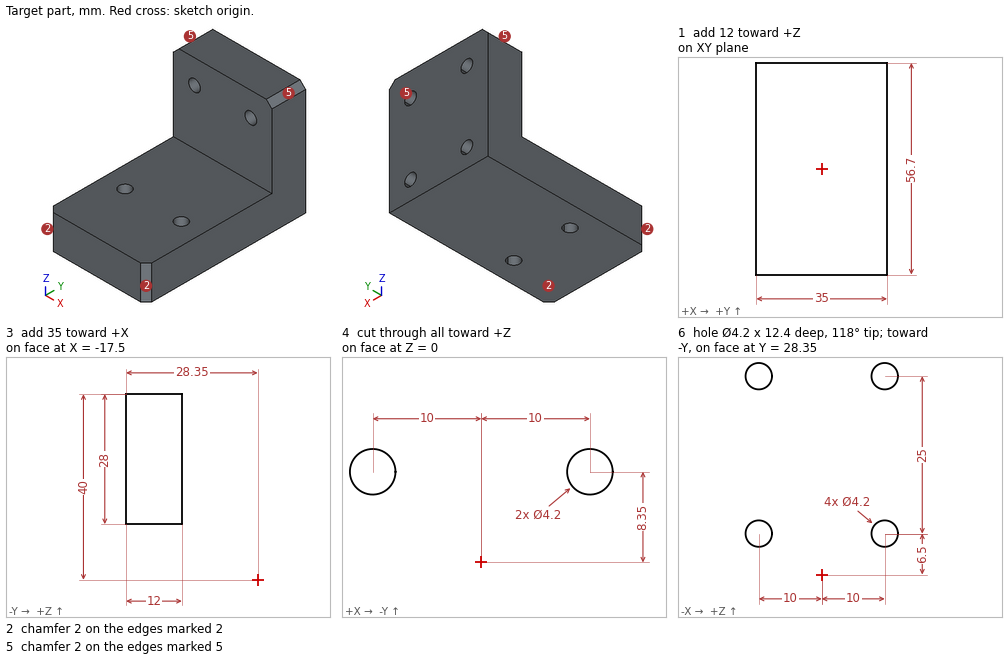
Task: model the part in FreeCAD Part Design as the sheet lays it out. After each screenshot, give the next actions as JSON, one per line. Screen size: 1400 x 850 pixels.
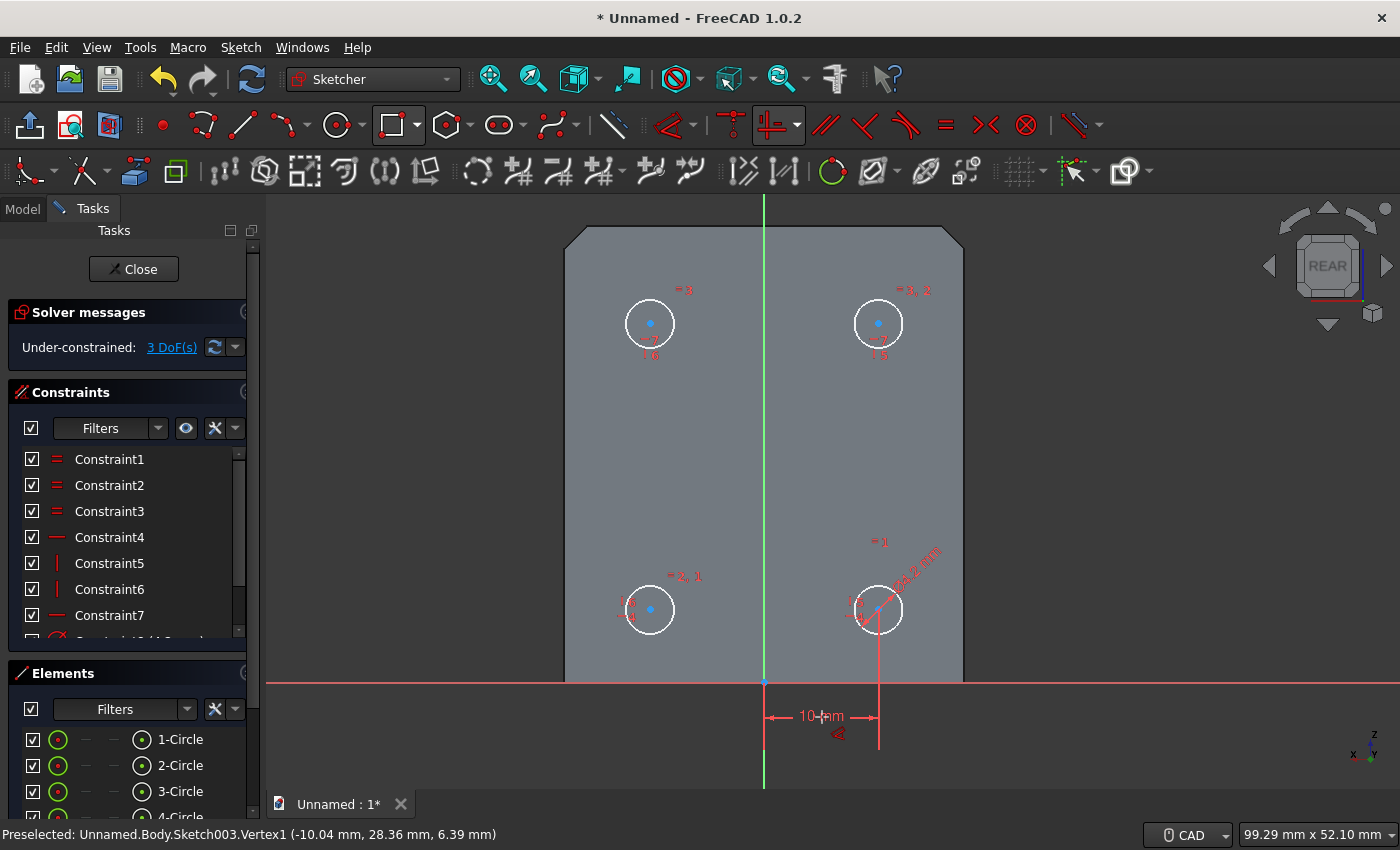
{"action": "left_click", "coordinate": [650, 610]}
{"action": "left_click", "coordinate": [707, 717]}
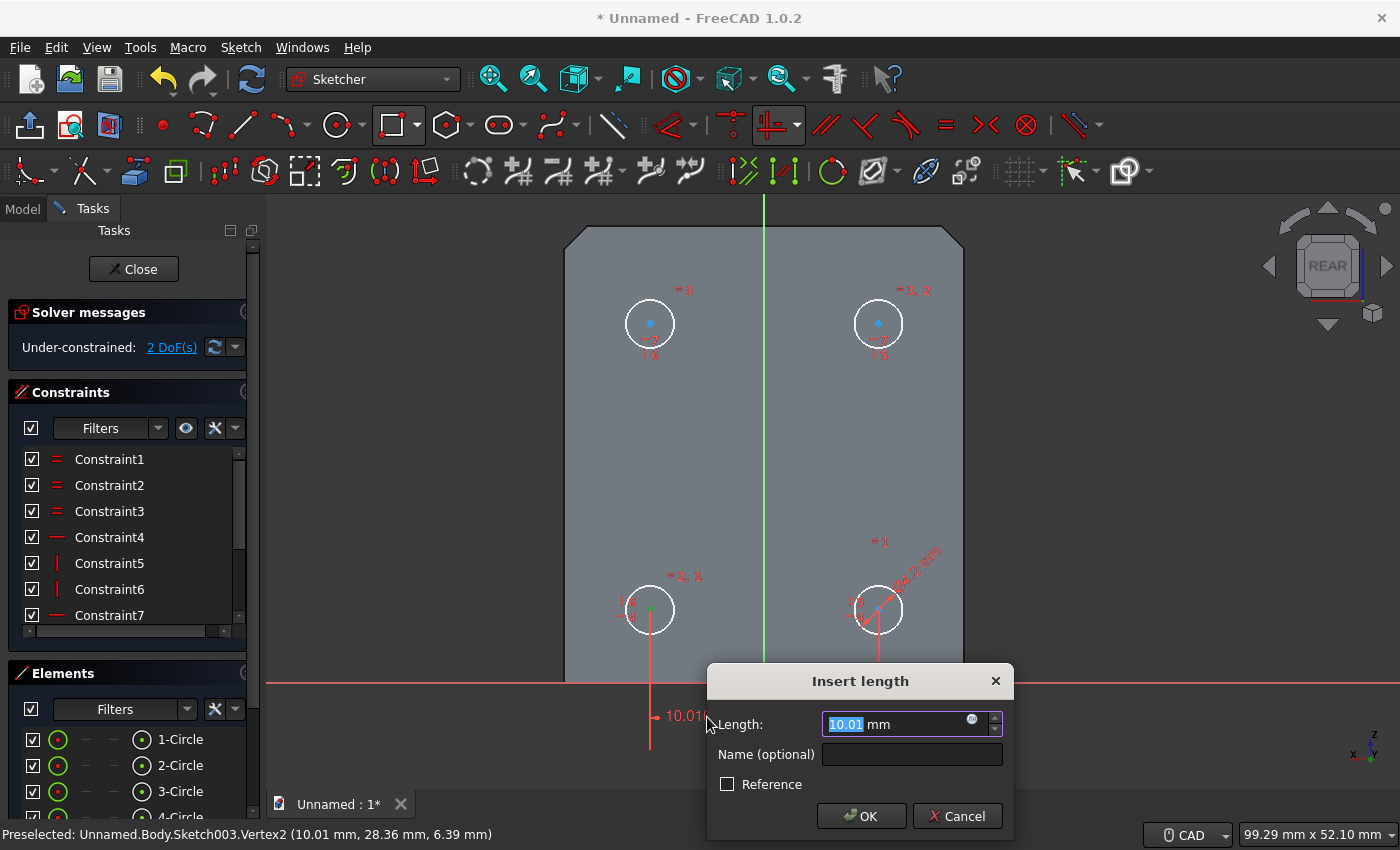
{"action": "type", "text": "10"}
{"action": "key", "text": "Return"}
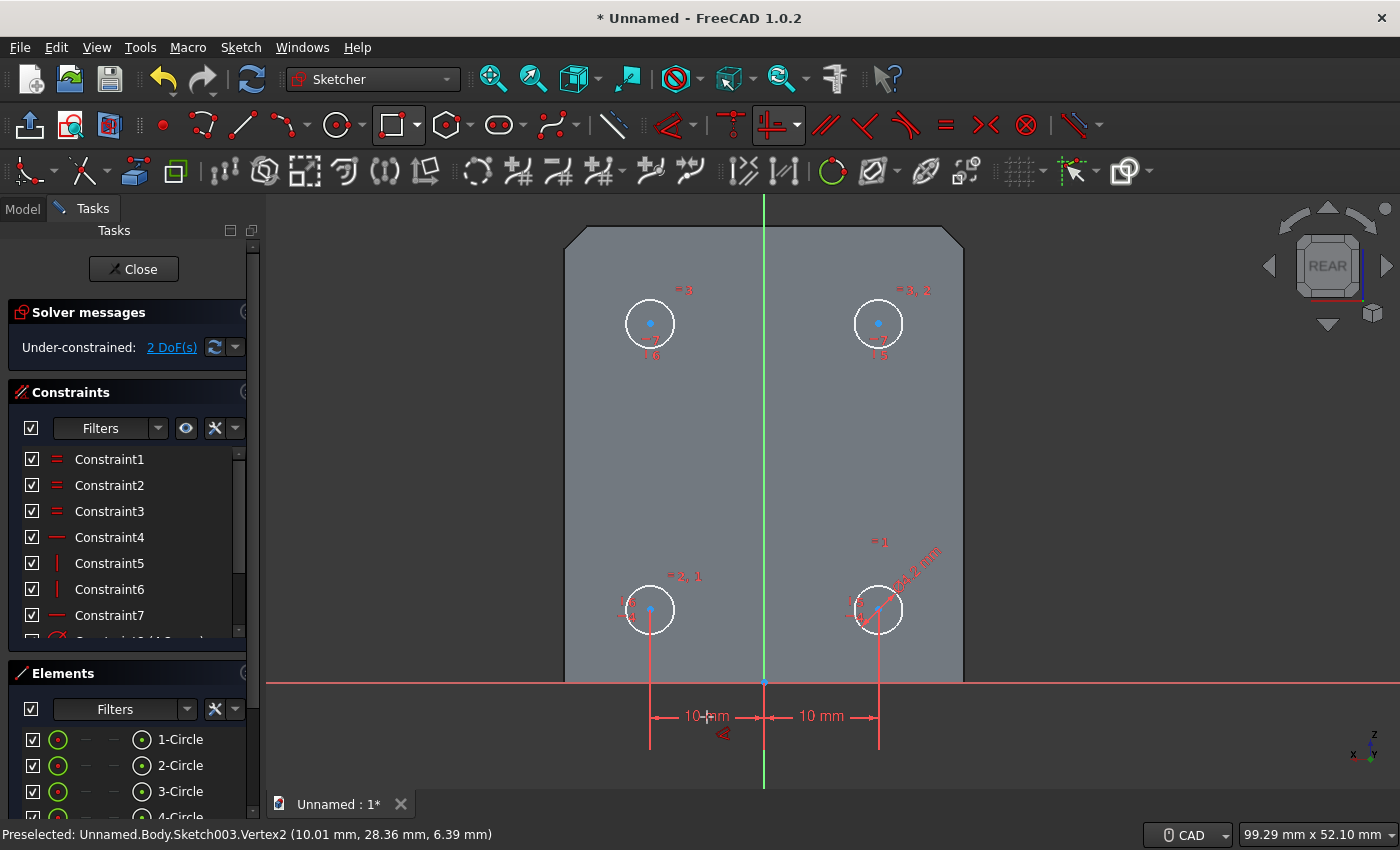
{"action": "left_click", "coordinate": [879, 610]}
{"action": "left_click", "coordinate": [913, 646]}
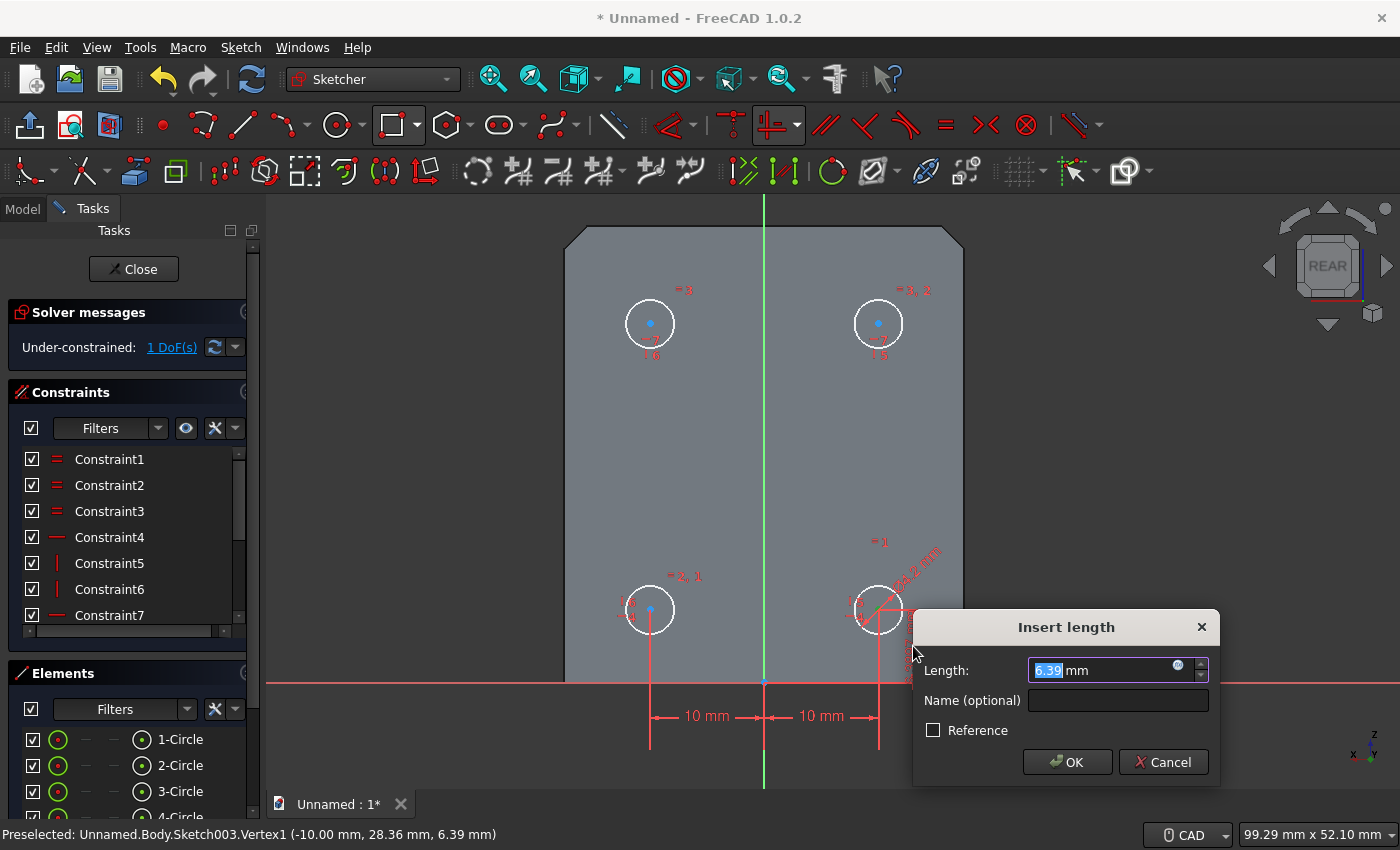
{"action": "type", "text": "6.5"}
{"action": "key", "text": "Return"}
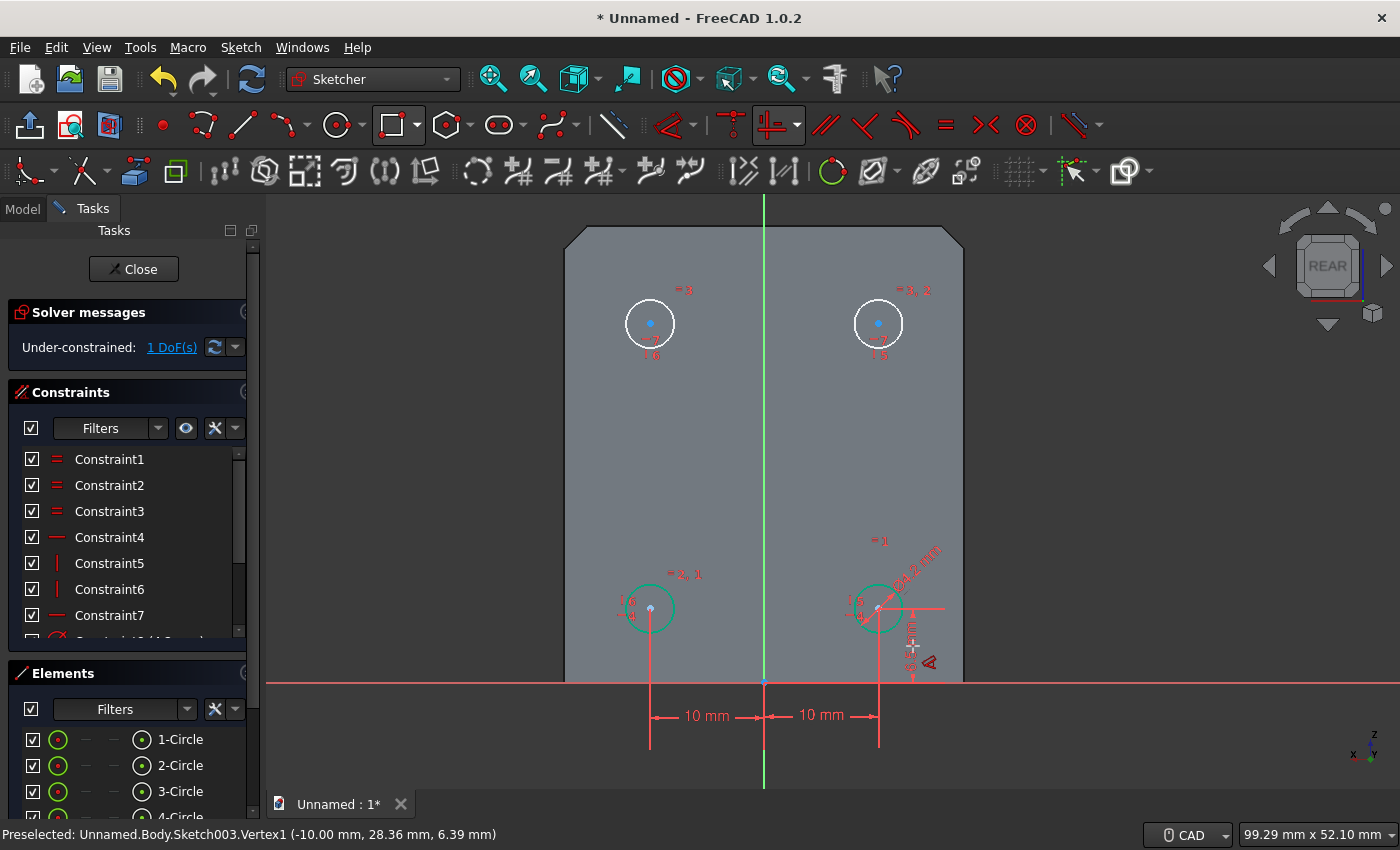
{"action": "left_click", "coordinate": [879, 609]}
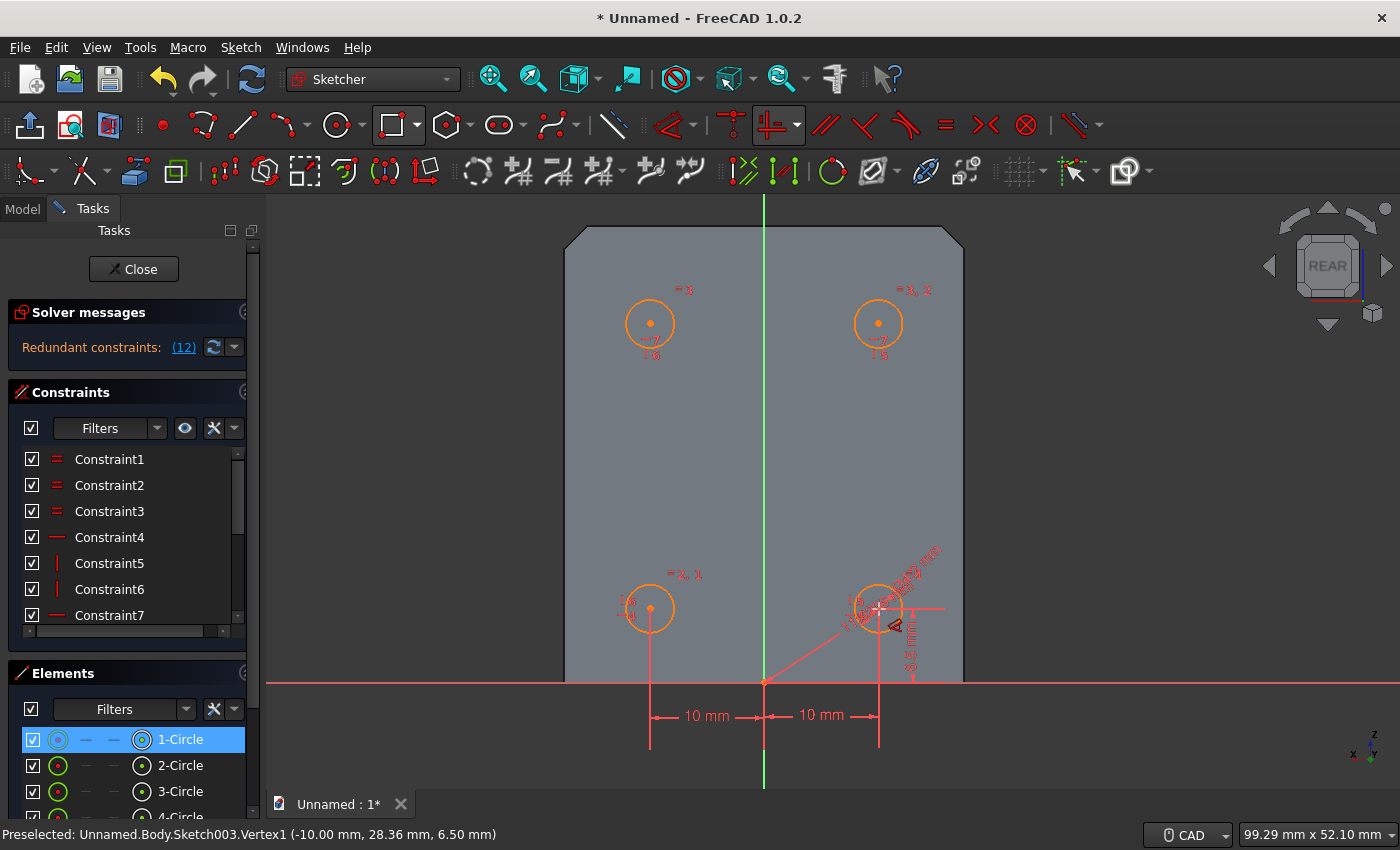
{"action": "left_click", "coordinate": [879, 324]}
{"action": "left_click", "coordinate": [913, 466]}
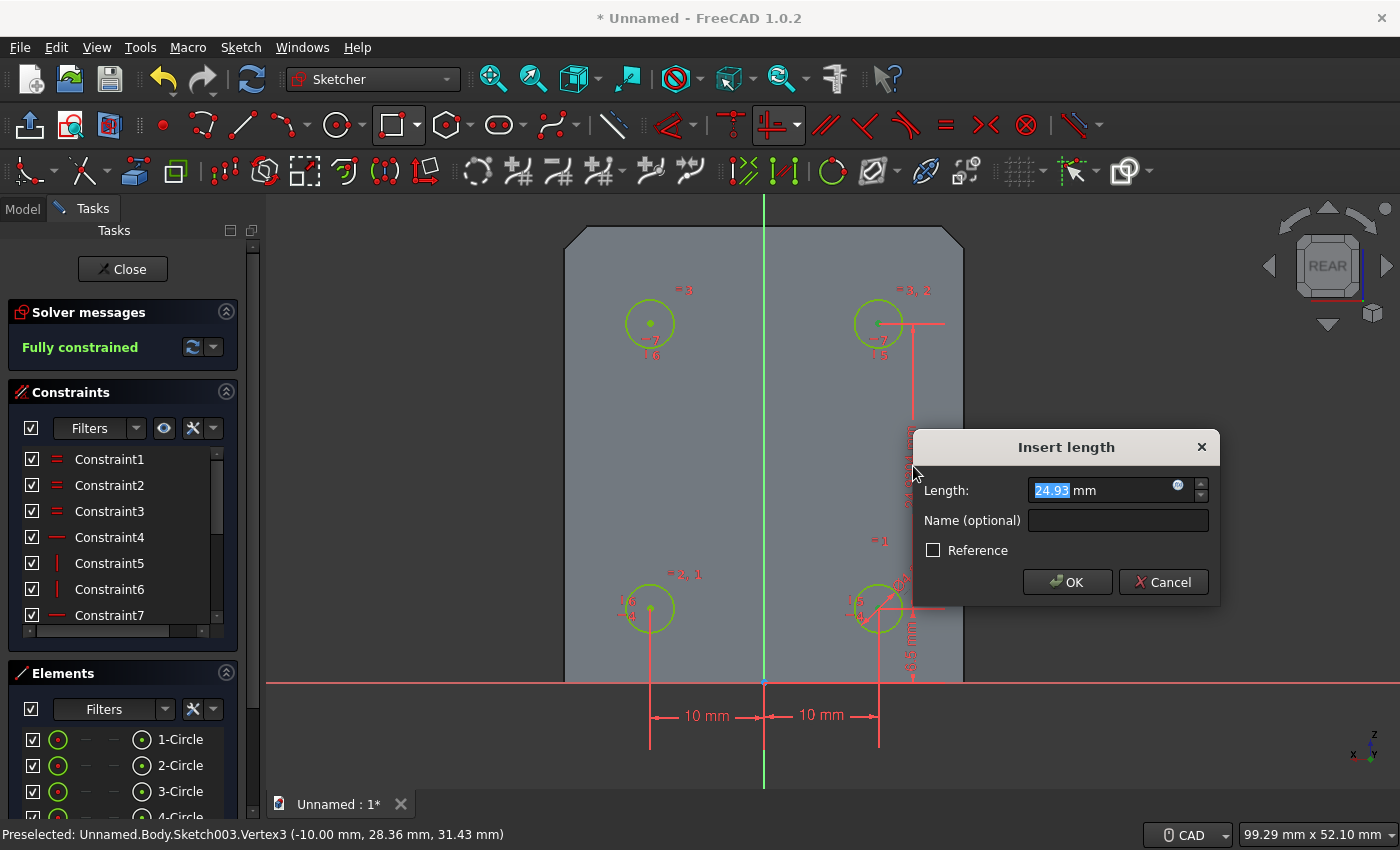
{"action": "type", "text": "25"}
{"action": "key", "text": "Return"}
{"action": "key", "text": "Escape"}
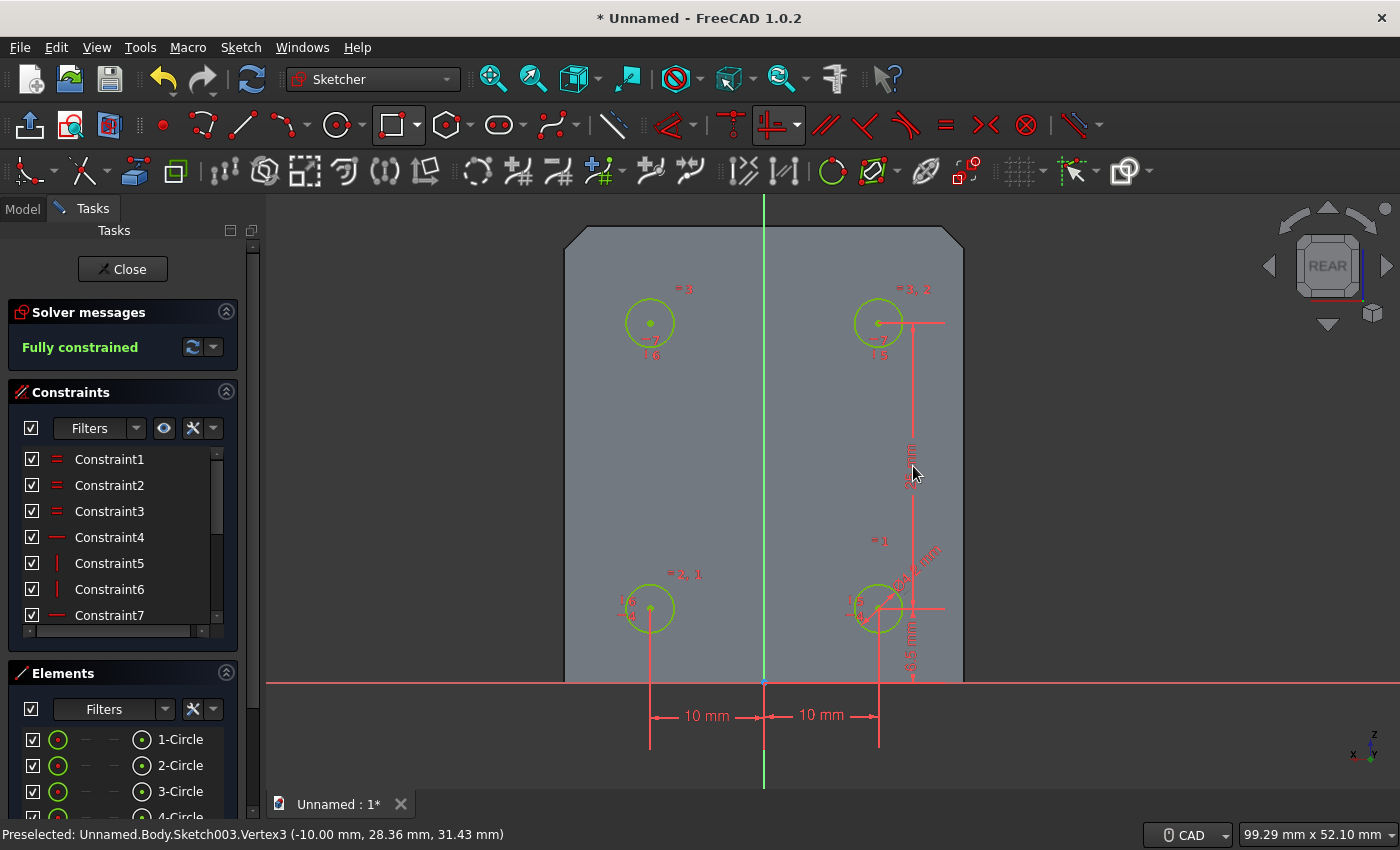
{"action": "left_click", "coordinate": [123, 269]}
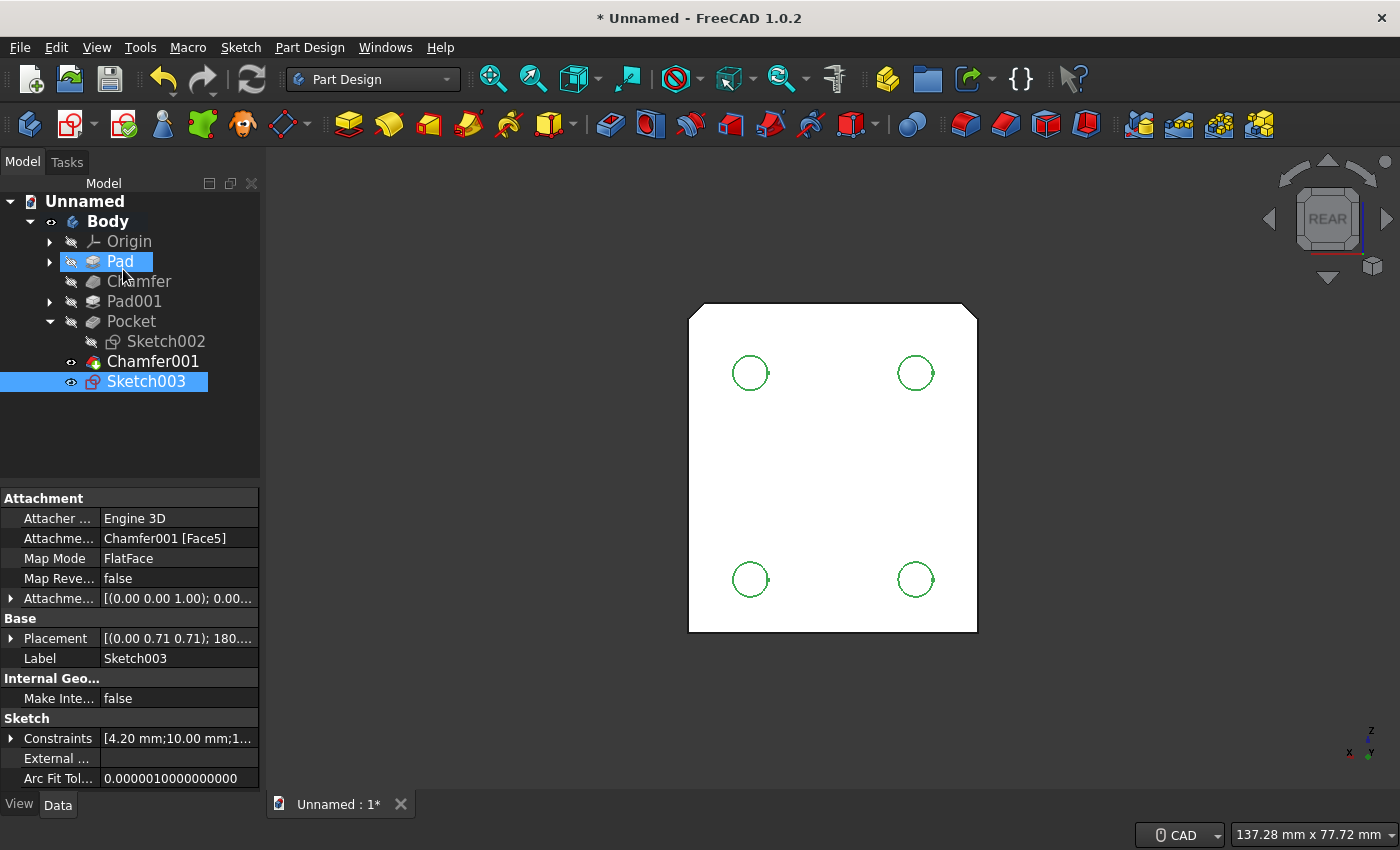
{"action": "left_click", "coordinate": [652, 124]}